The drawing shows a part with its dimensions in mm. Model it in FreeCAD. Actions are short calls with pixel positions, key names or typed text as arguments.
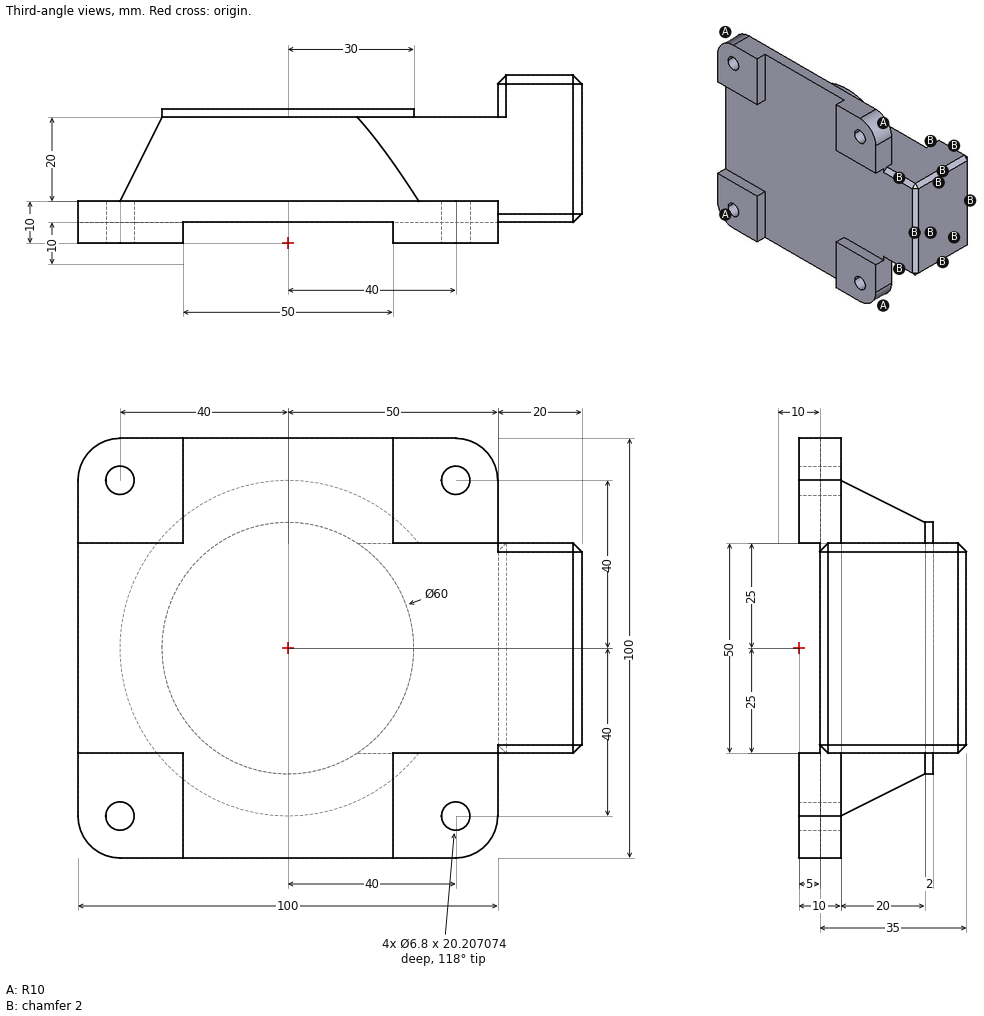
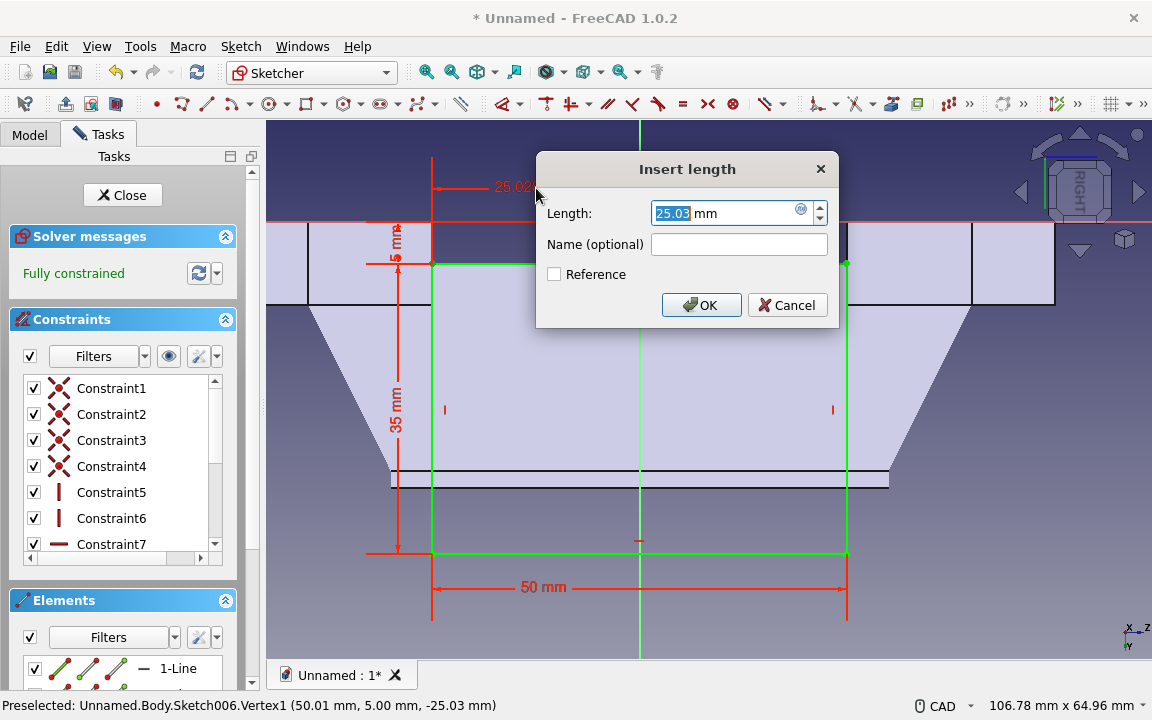
text(25)
key(Return)
key(Escape)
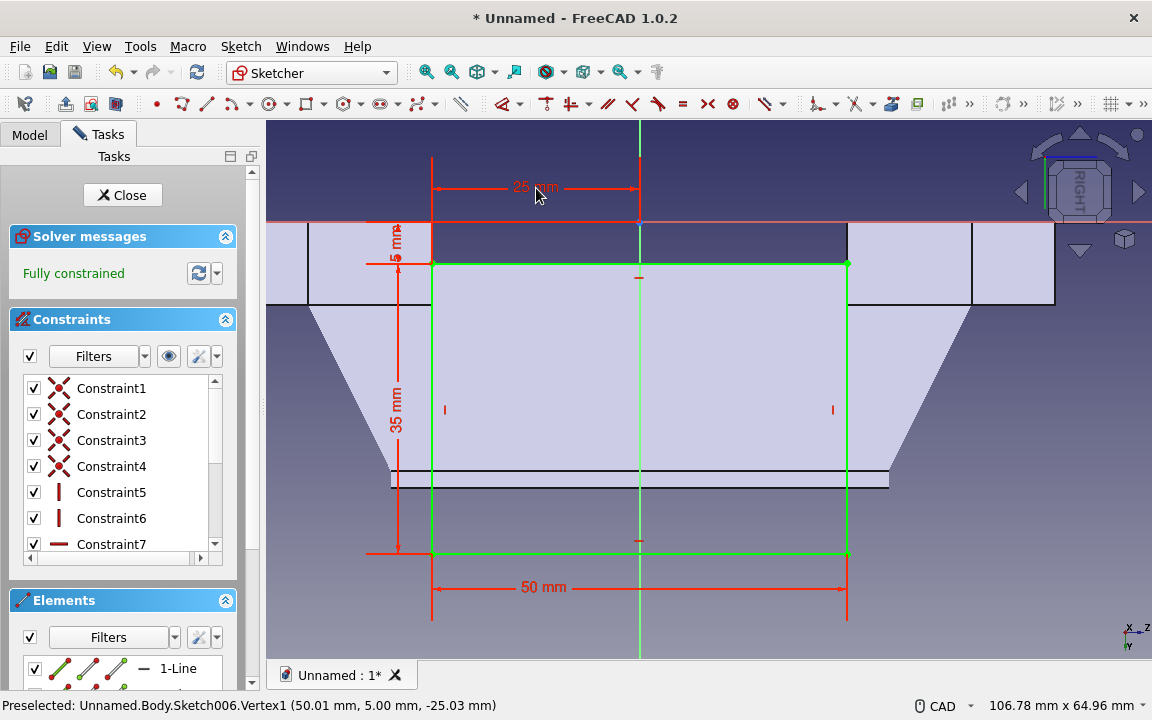
click(123, 195)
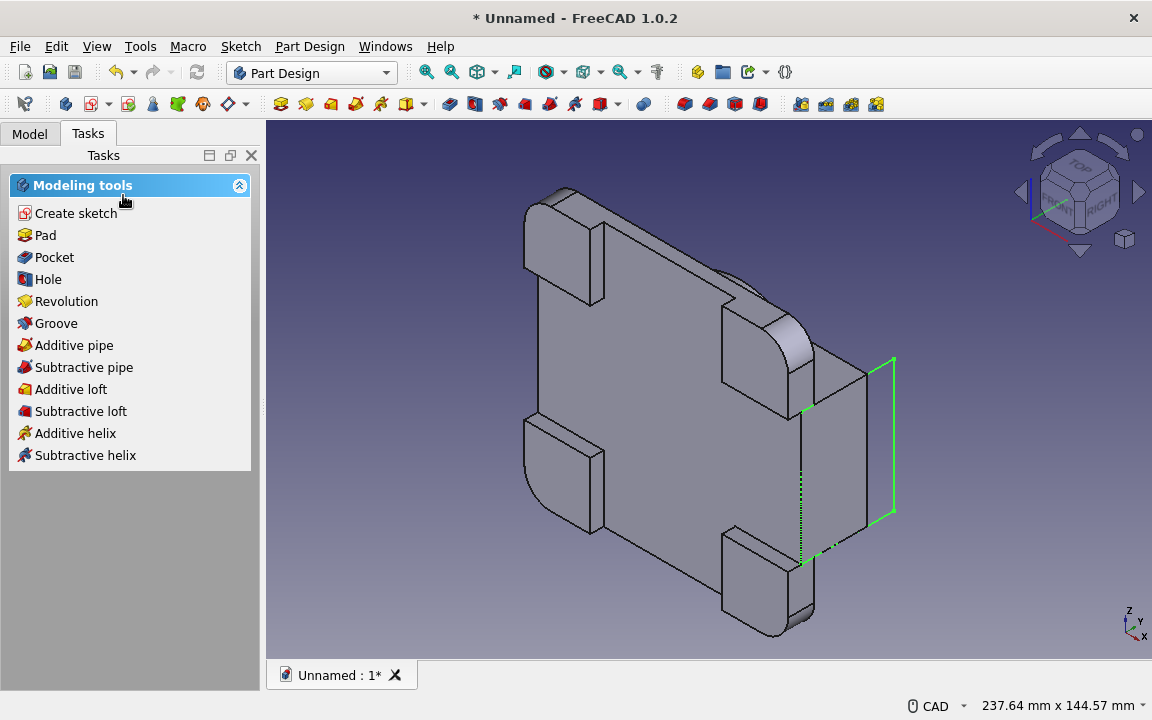
click(281, 104)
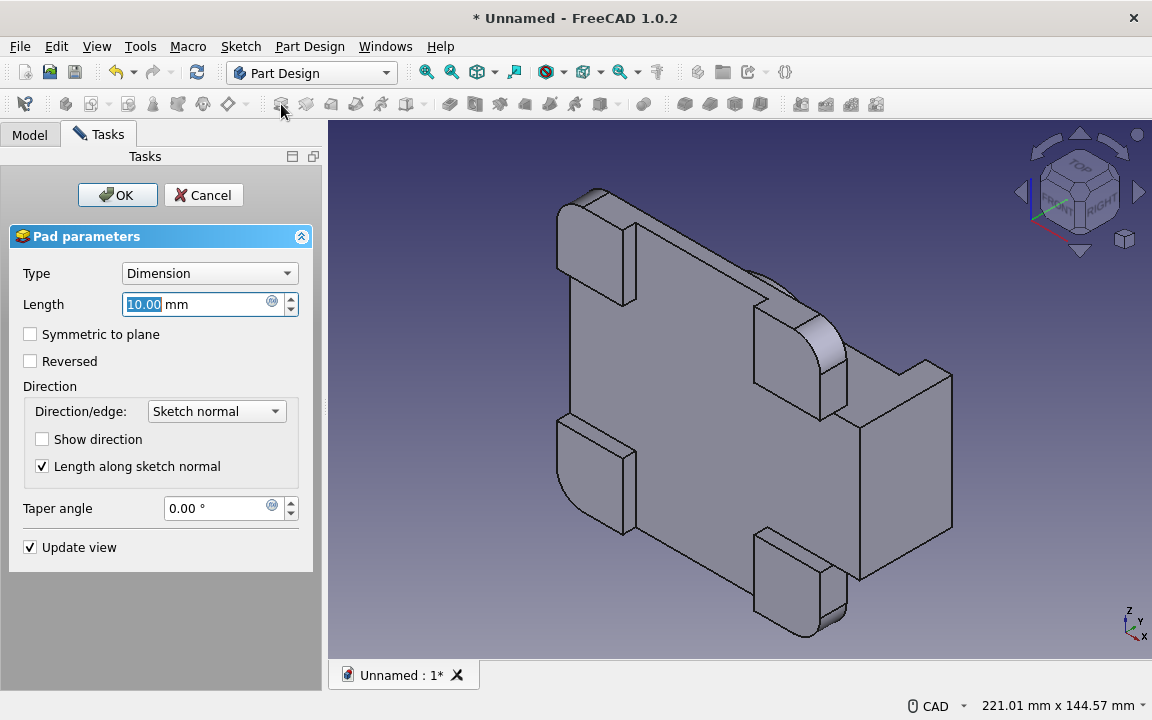
text(20)
key(Tab)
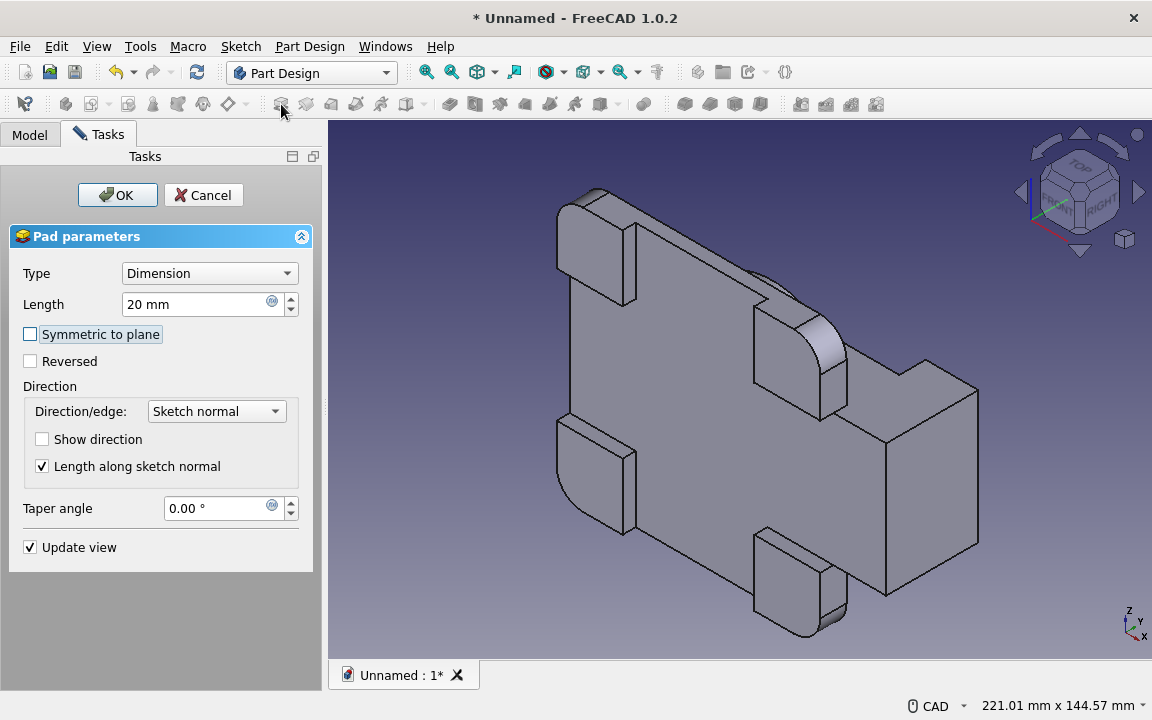
click(118, 195)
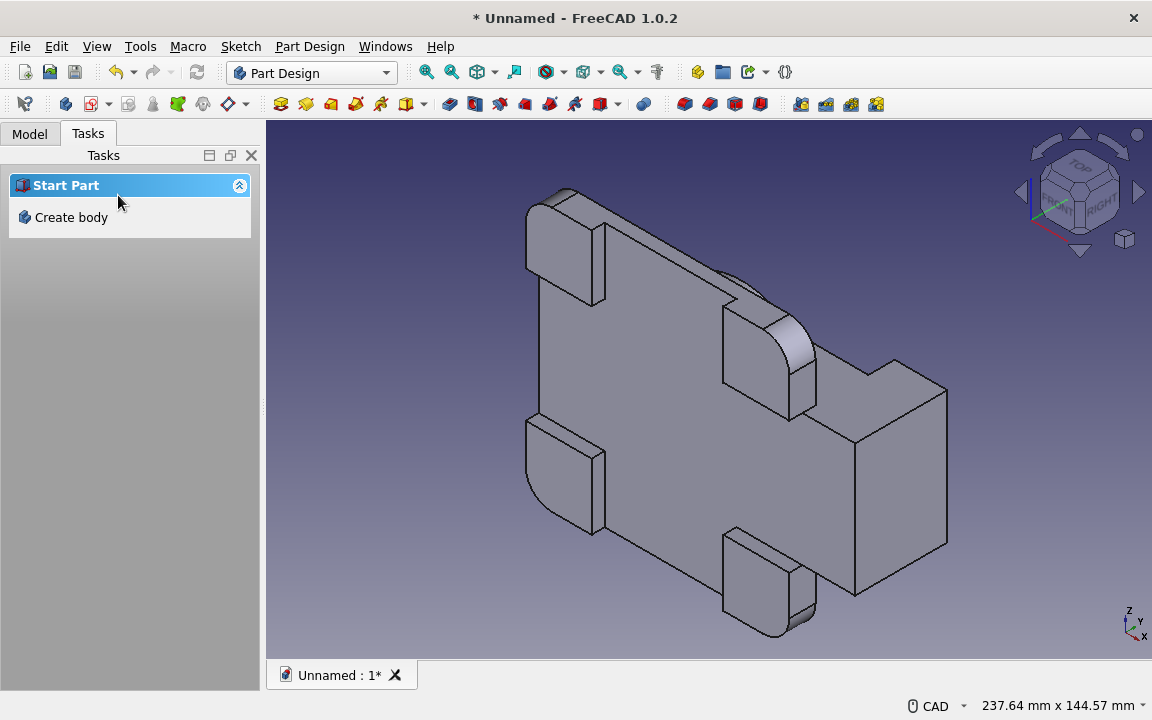
click(427, 72)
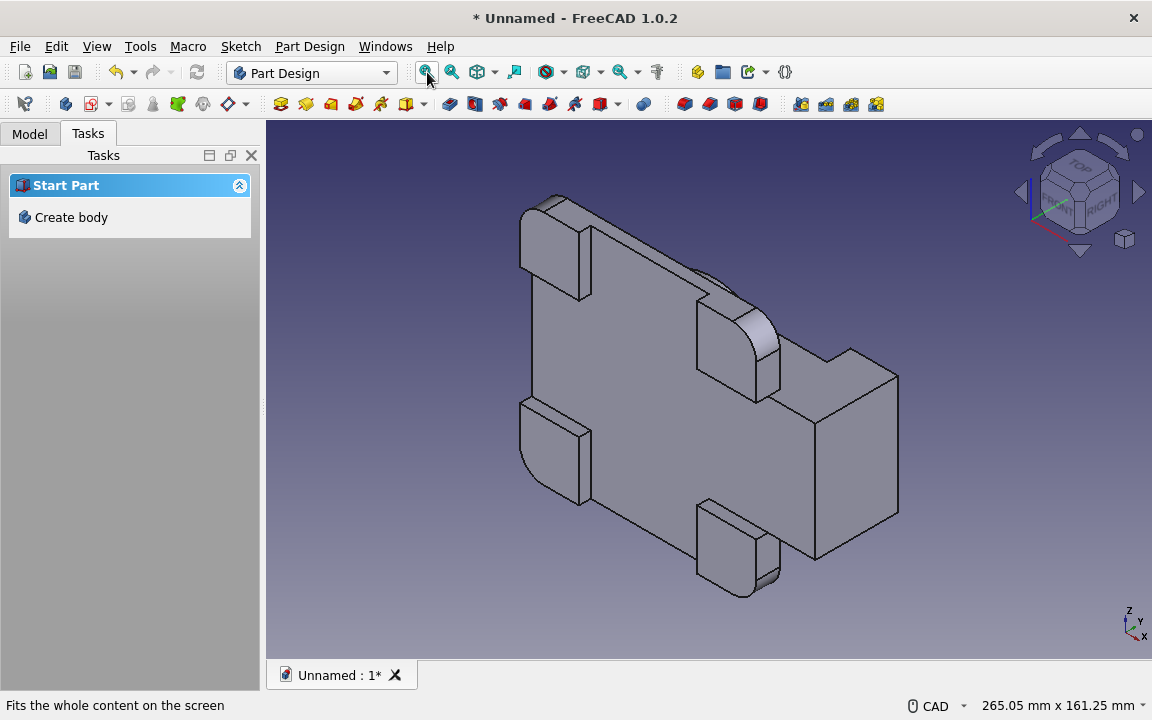
click(857, 447)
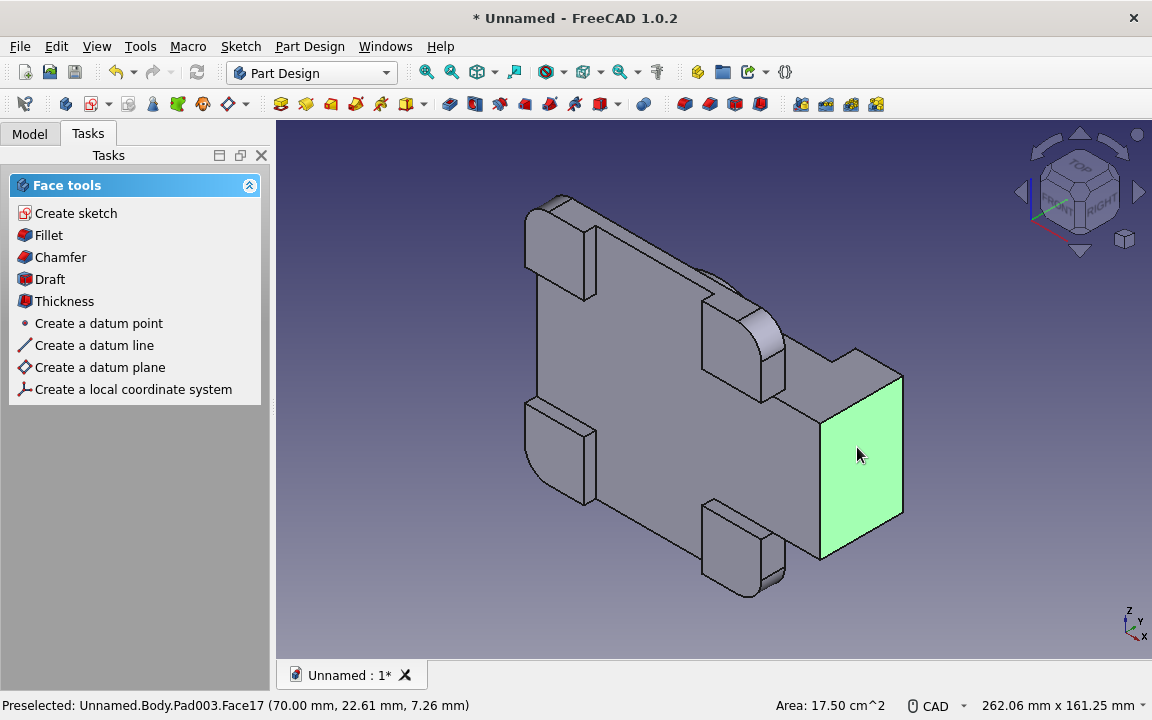
click(797, 409, ctrl)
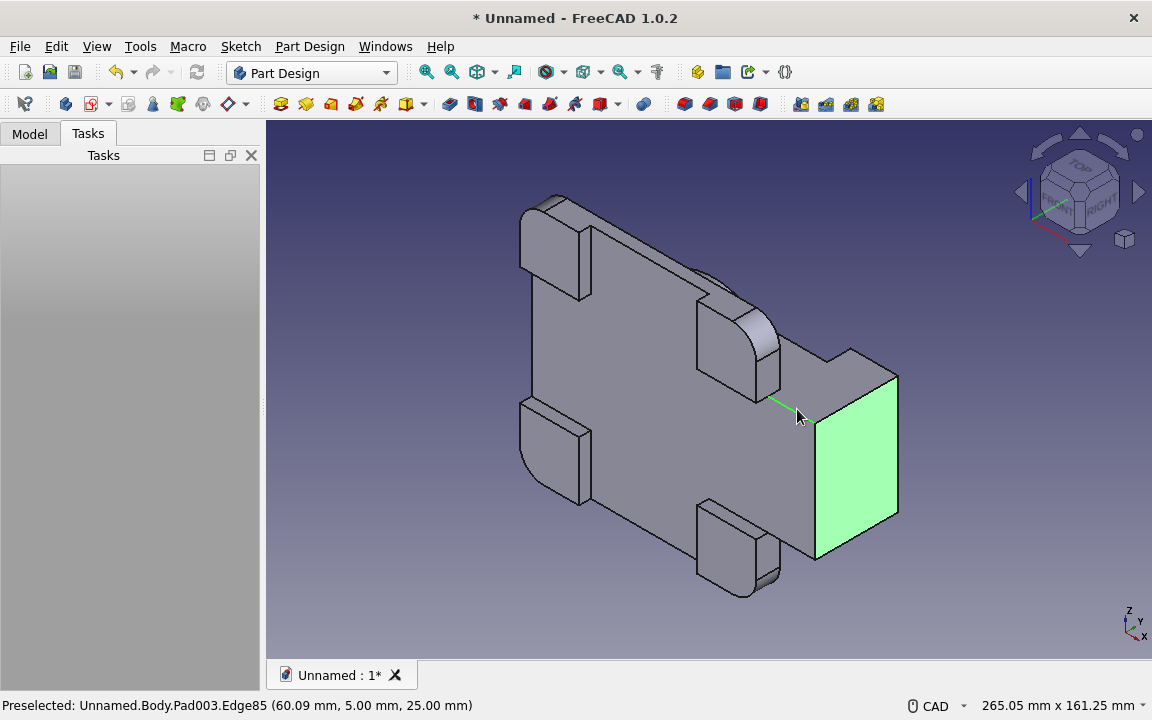
key(2)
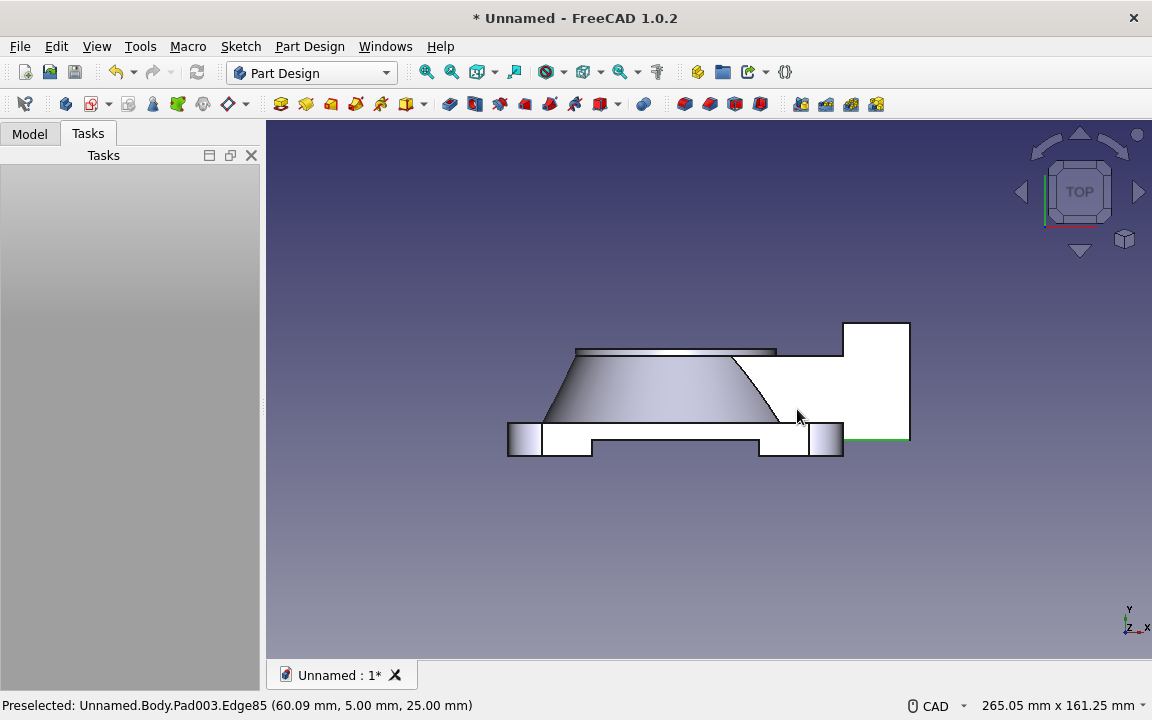
click(843, 338, ctrl)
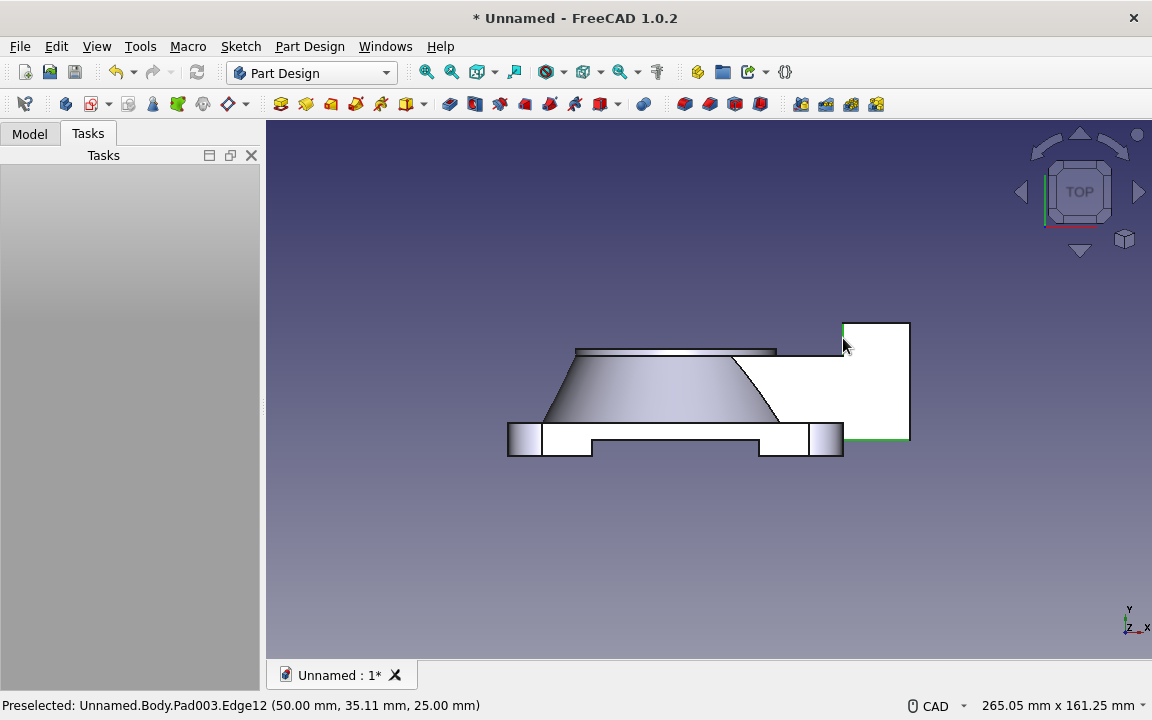
key(0)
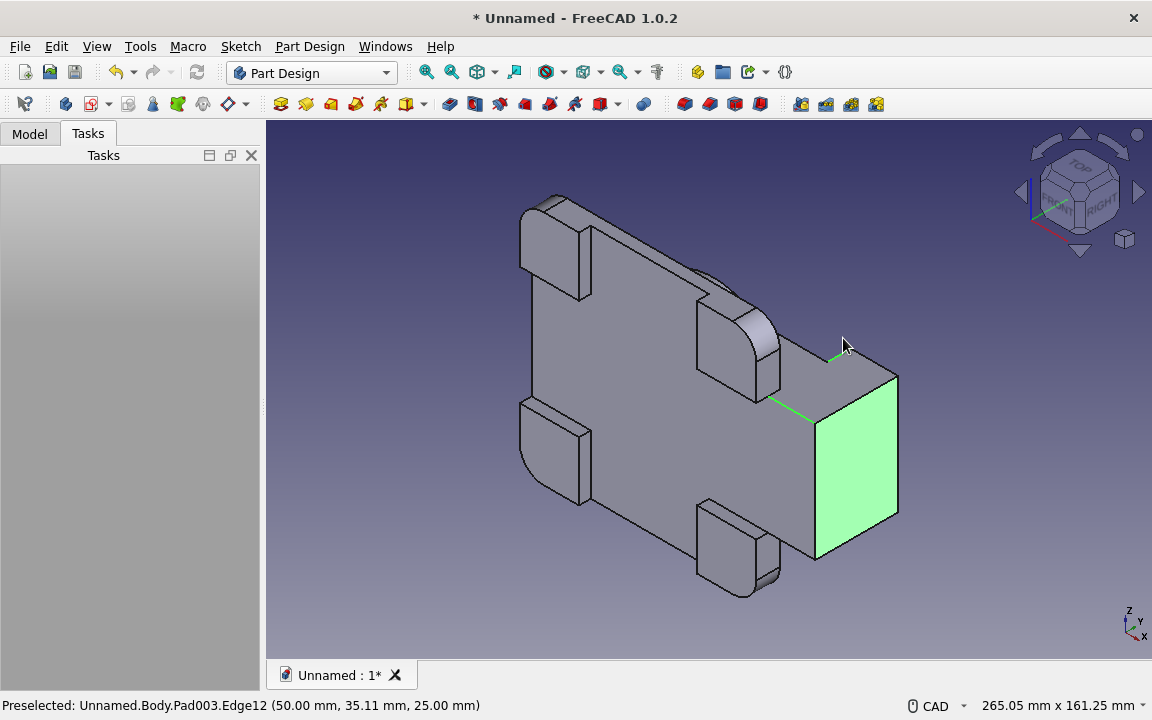
key(1)